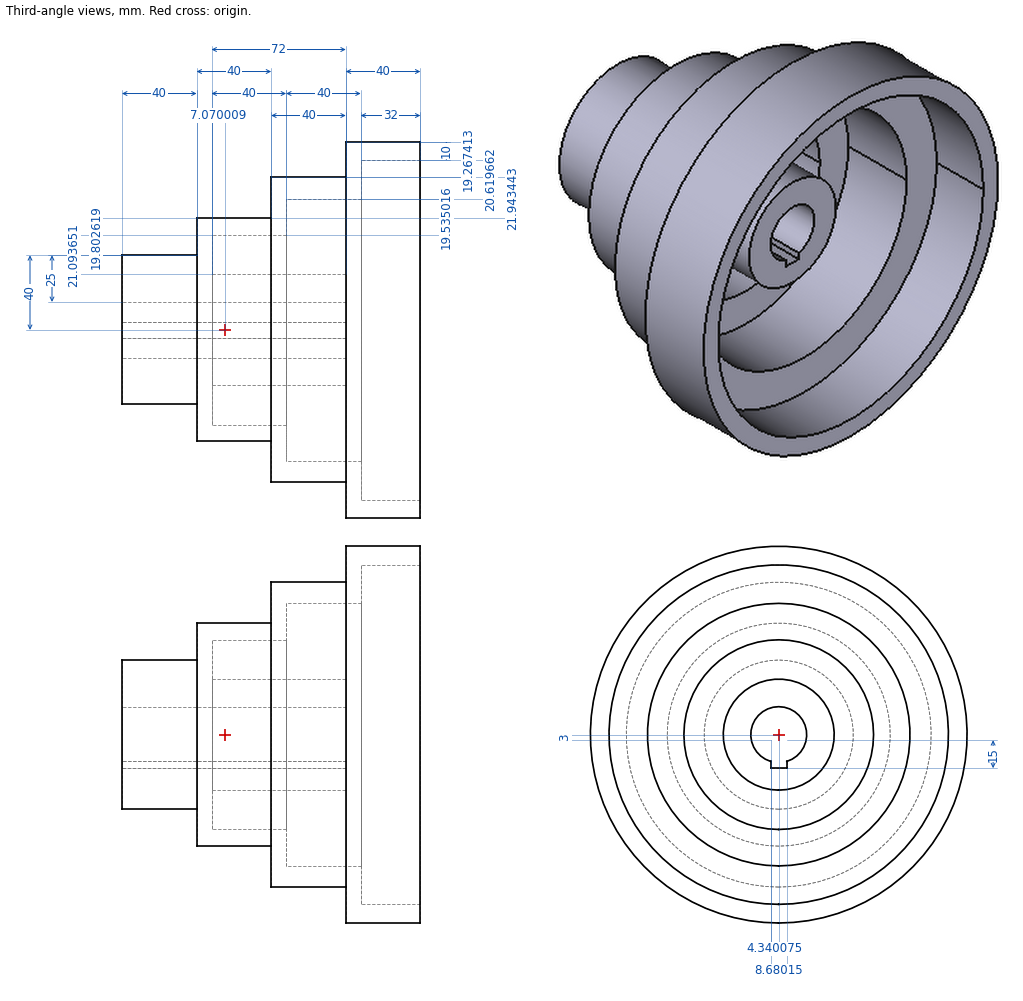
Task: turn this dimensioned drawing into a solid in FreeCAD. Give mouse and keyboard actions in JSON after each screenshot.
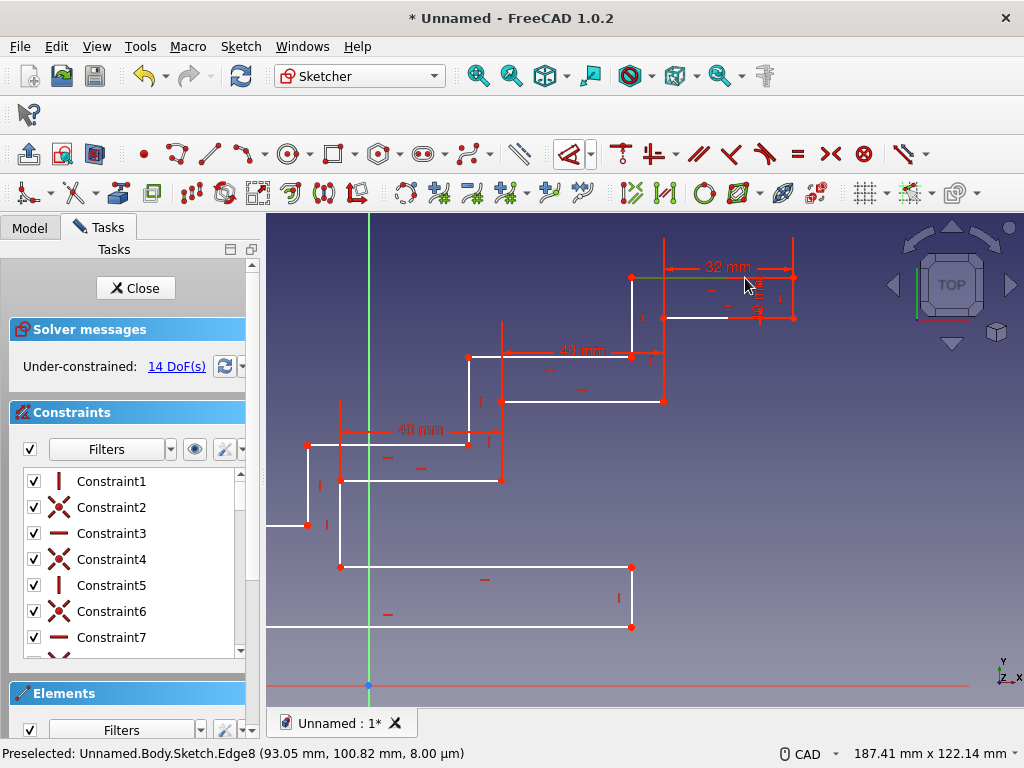
{"action": "left_click", "coordinate": [590, 154]}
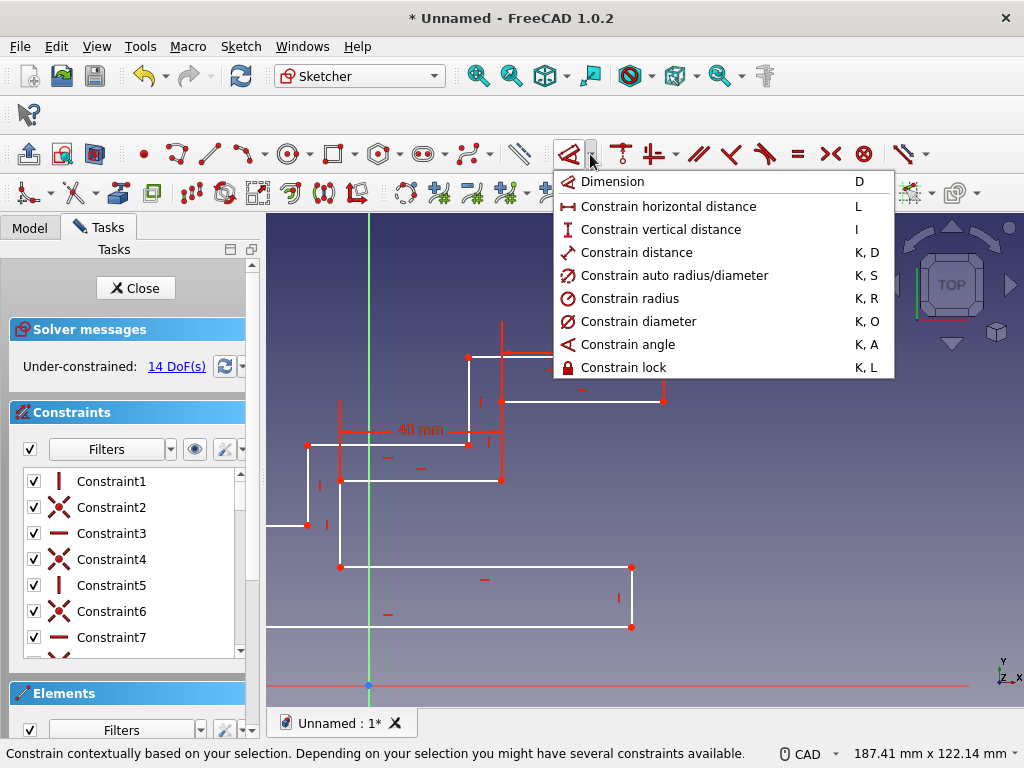
{"action": "left_click", "coordinate": [724, 206]}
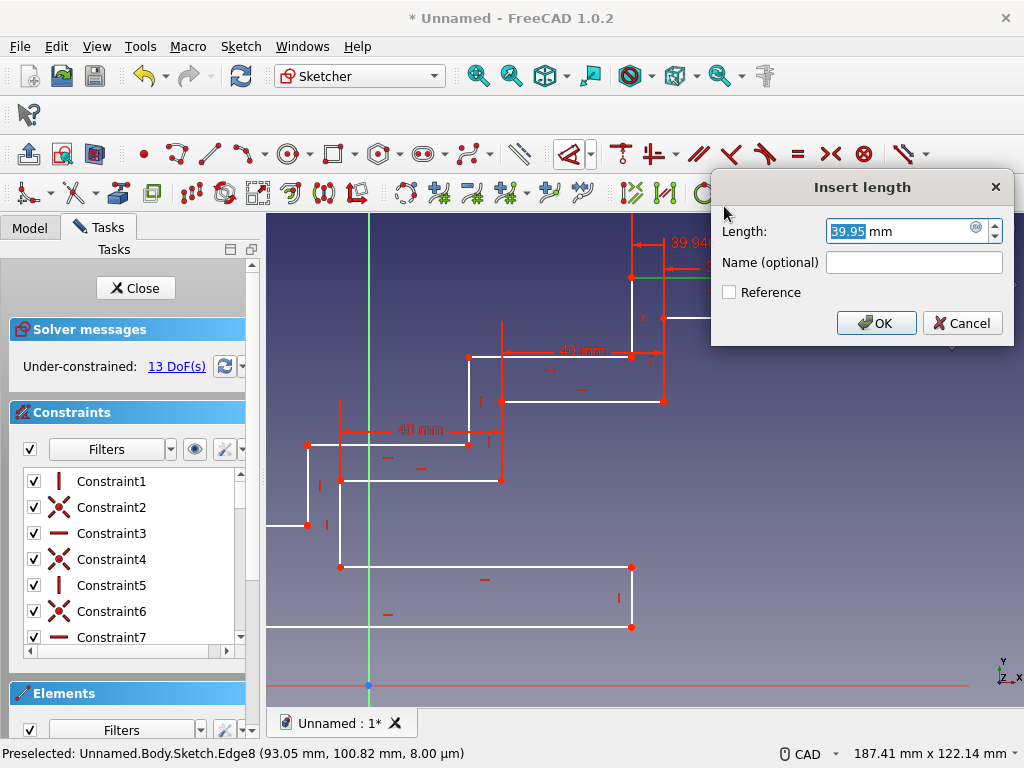
{"action": "type", "text": "40"}
{"action": "key", "text": "Return"}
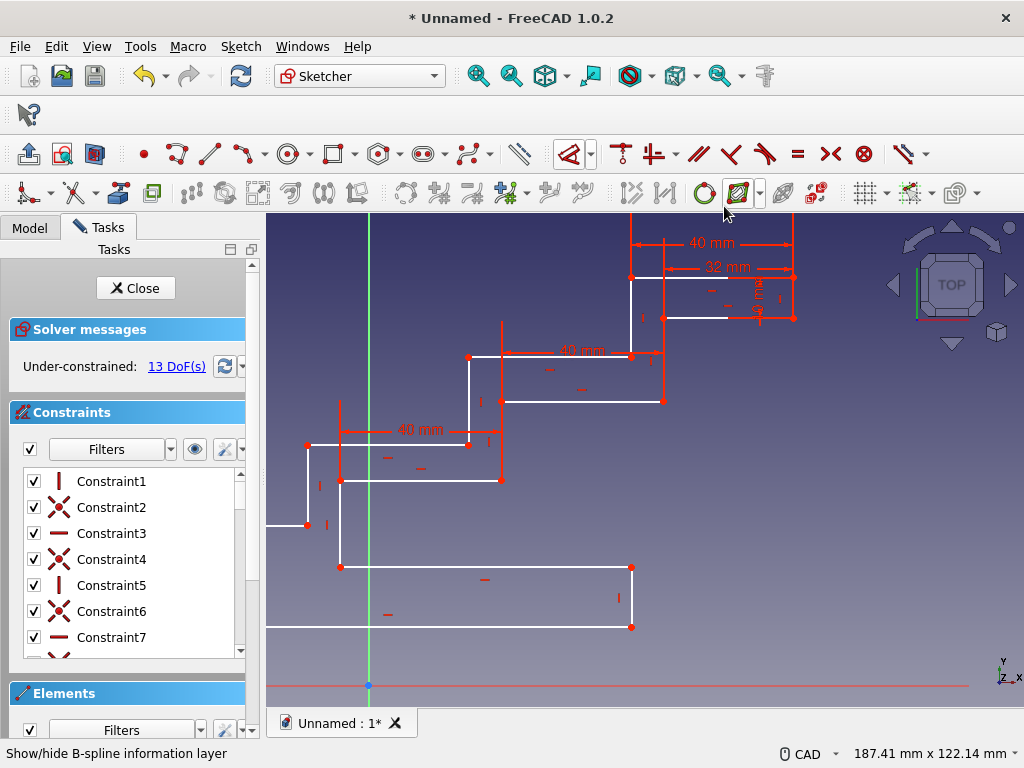
{"action": "left_click", "coordinate": [518, 357]}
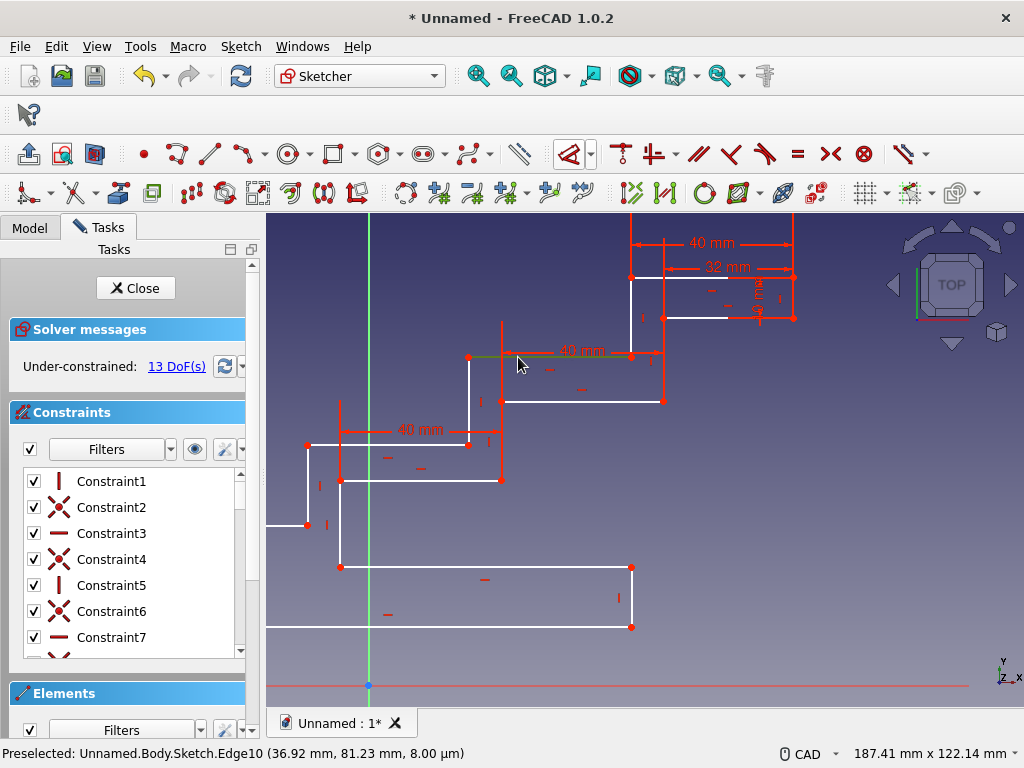
{"action": "left_click", "coordinate": [590, 154]}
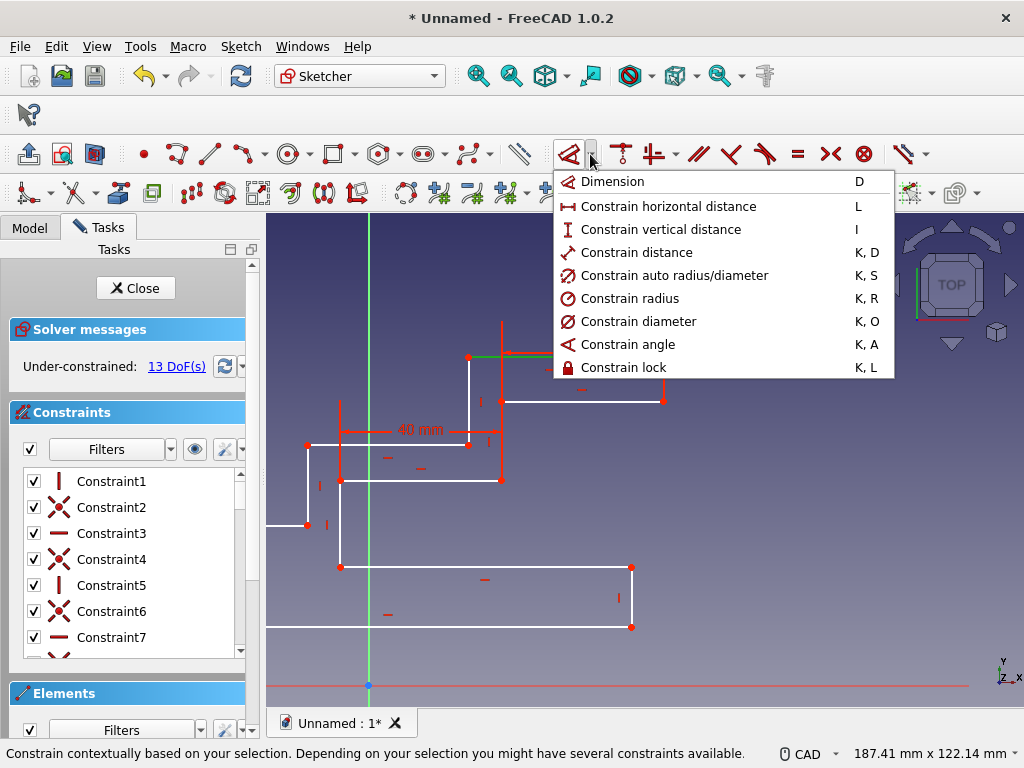
{"action": "left_click", "coordinate": [724, 206]}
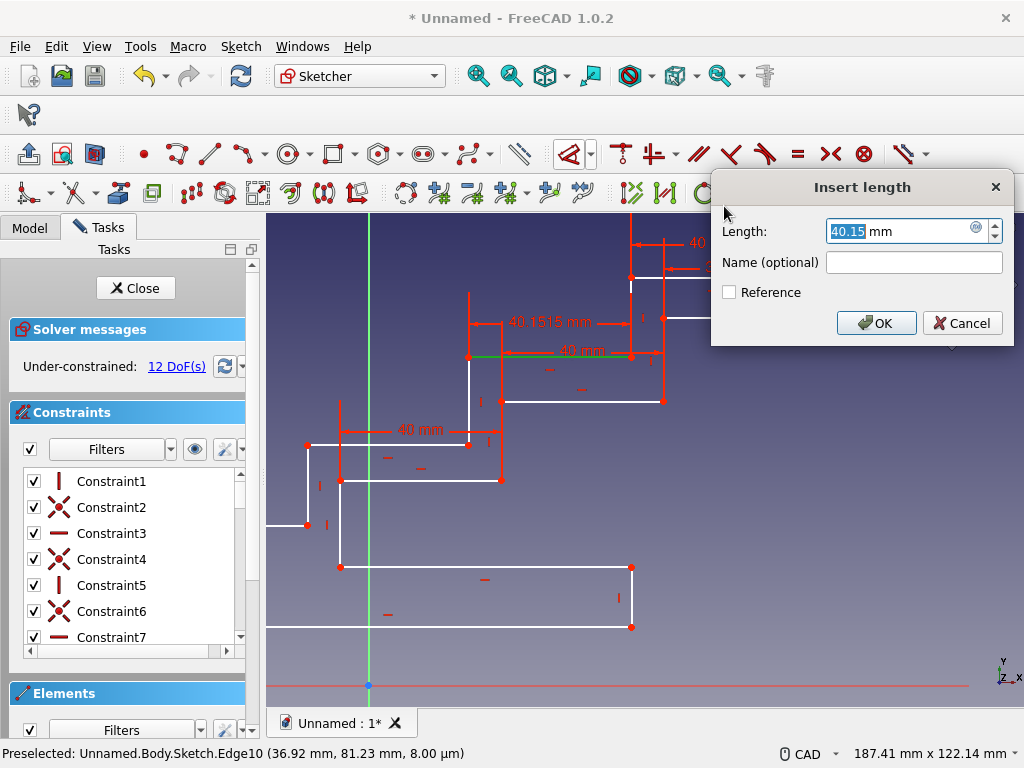
{"action": "type", "text": "40"}
{"action": "key", "text": "Return"}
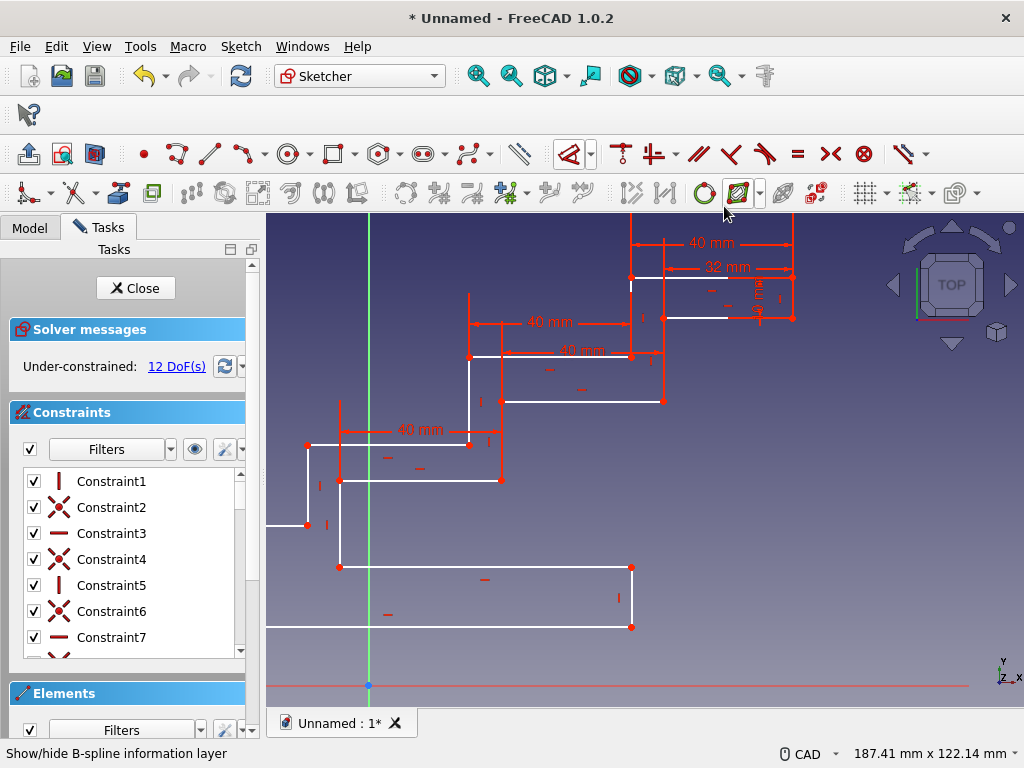
{"action": "left_click", "coordinate": [421, 445]}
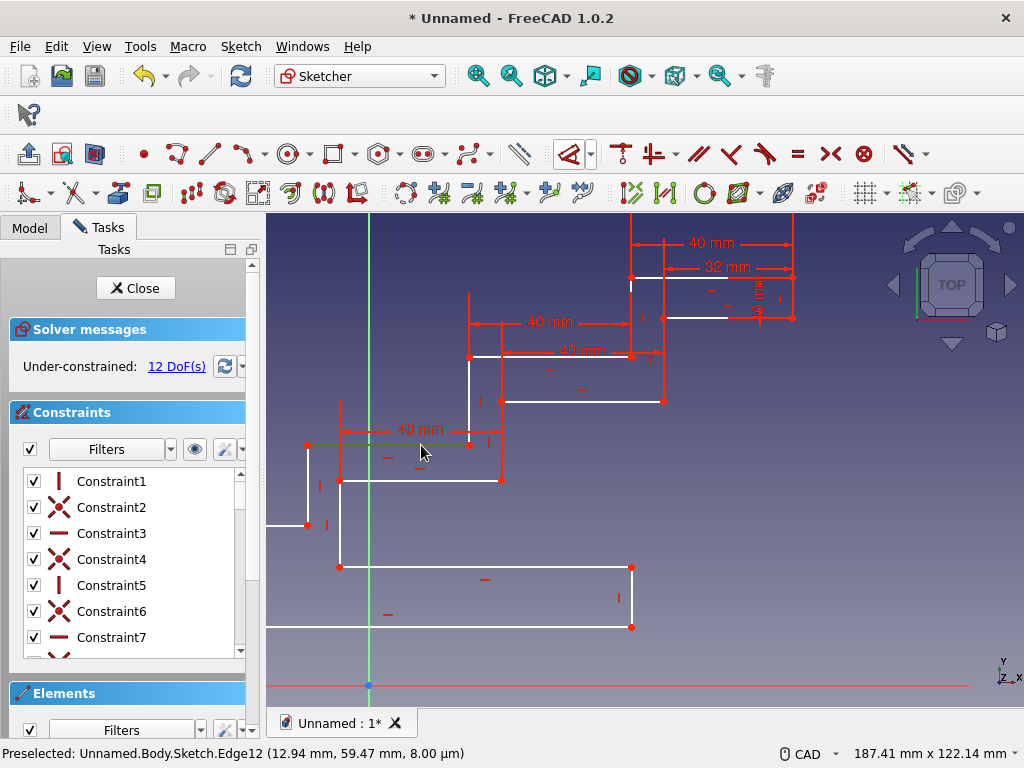
{"action": "key", "text": "l"}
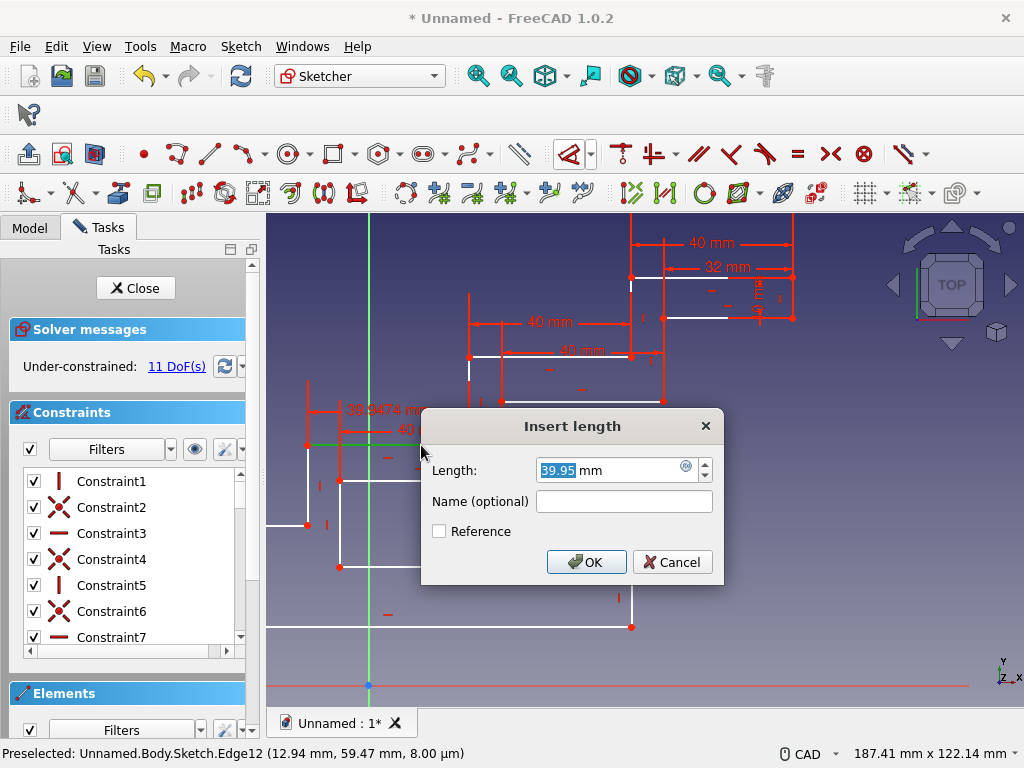
{"action": "type", "text": "40"}
{"action": "key", "text": "Return"}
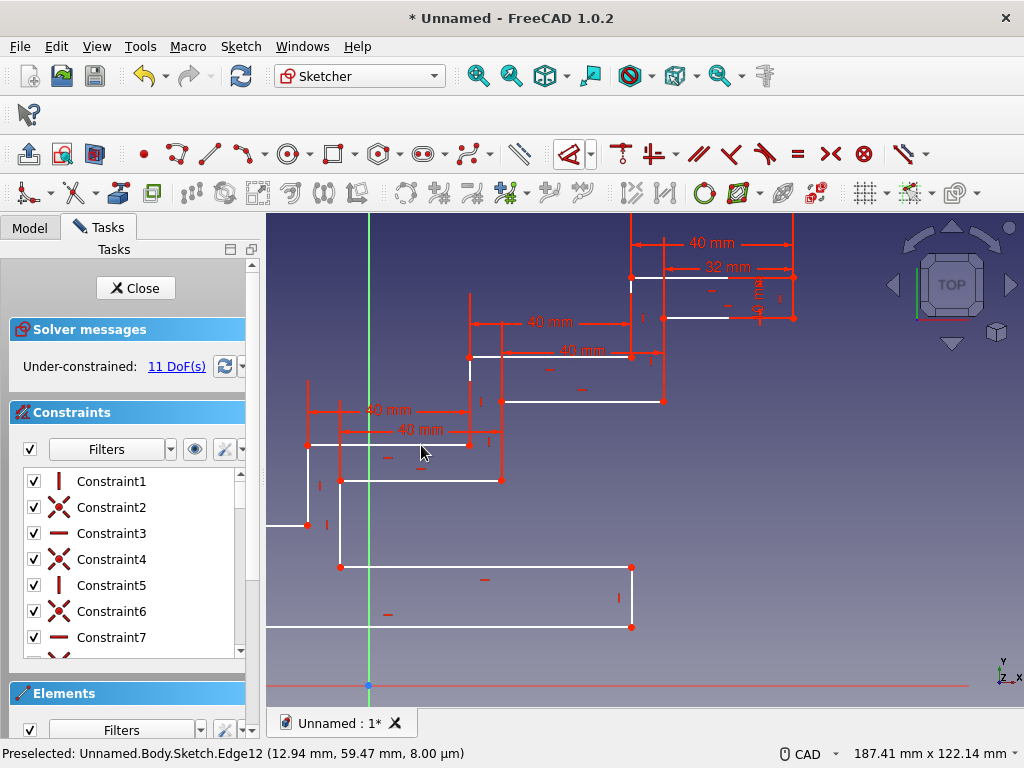
{"action": "scroll", "coordinate": [794, 417], "scroll_direction": "down", "scroll_amount": 2}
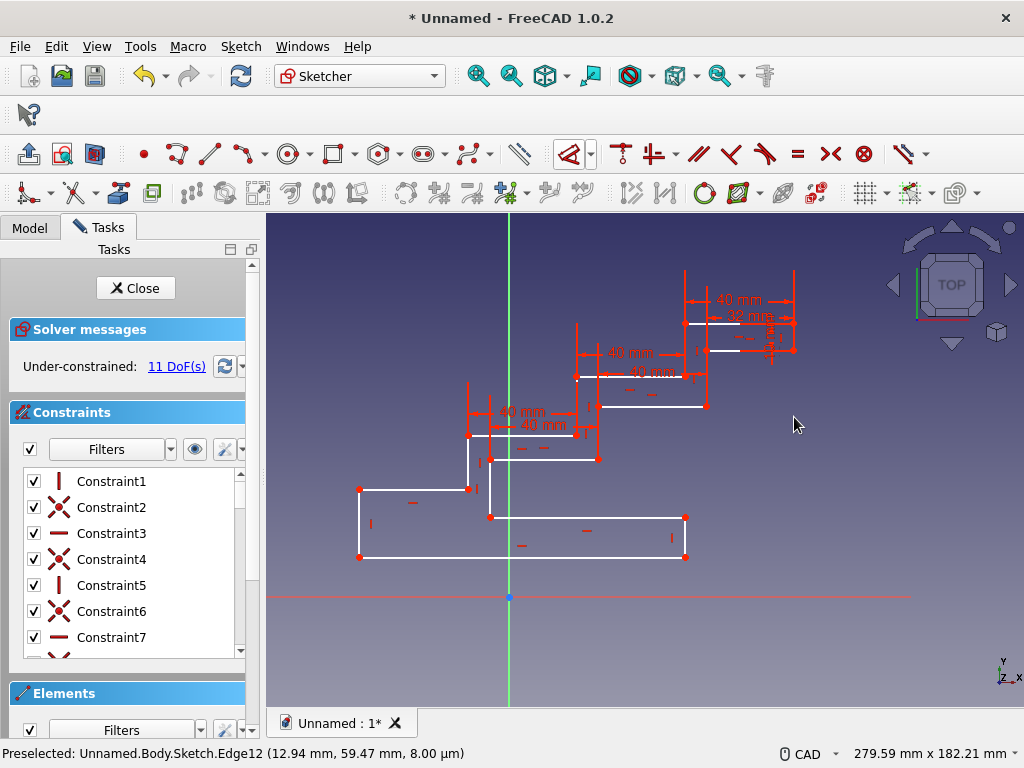
{"action": "left_click", "coordinate": [436, 490]}